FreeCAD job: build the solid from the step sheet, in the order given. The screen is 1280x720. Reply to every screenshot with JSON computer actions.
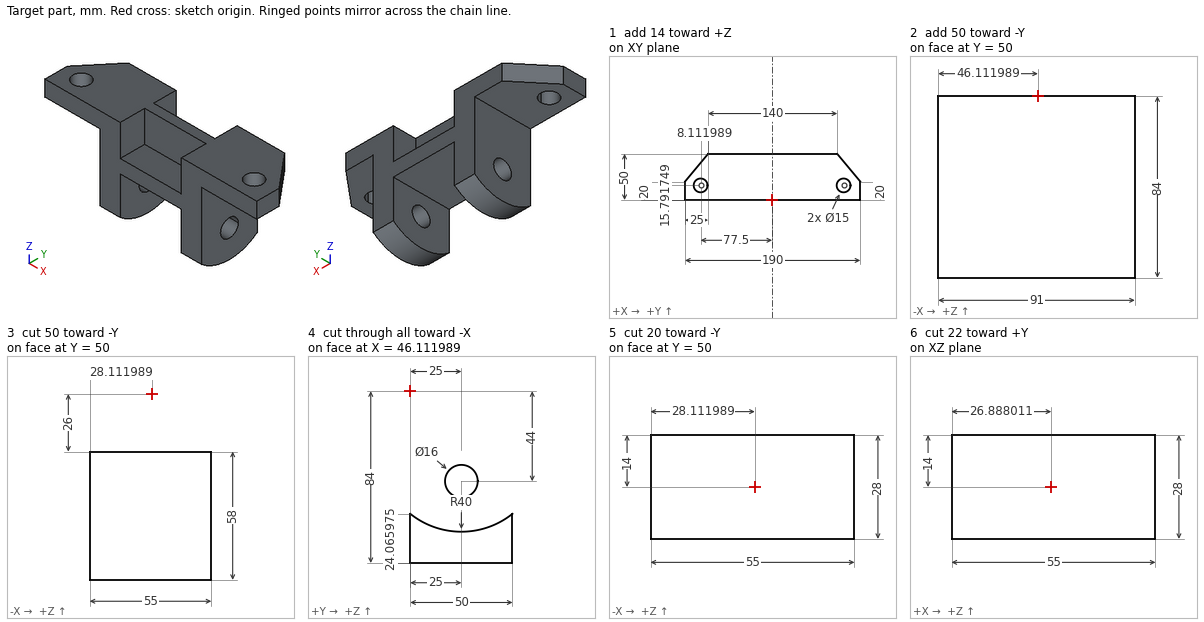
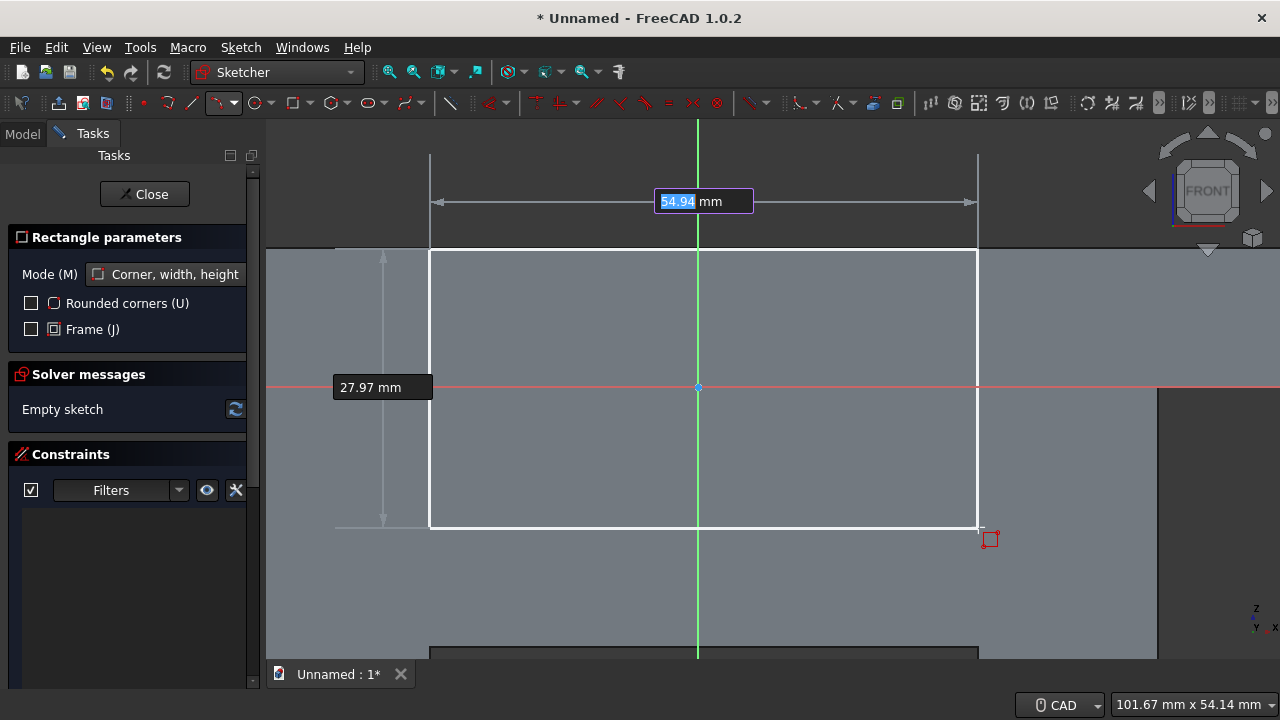
{"action": "type", "text": "55"}
{"action": "key", "text": "Tab"}
{"action": "type", "text": "28"}
{"action": "key", "text": "Return"}
{"action": "key", "text": "Escape"}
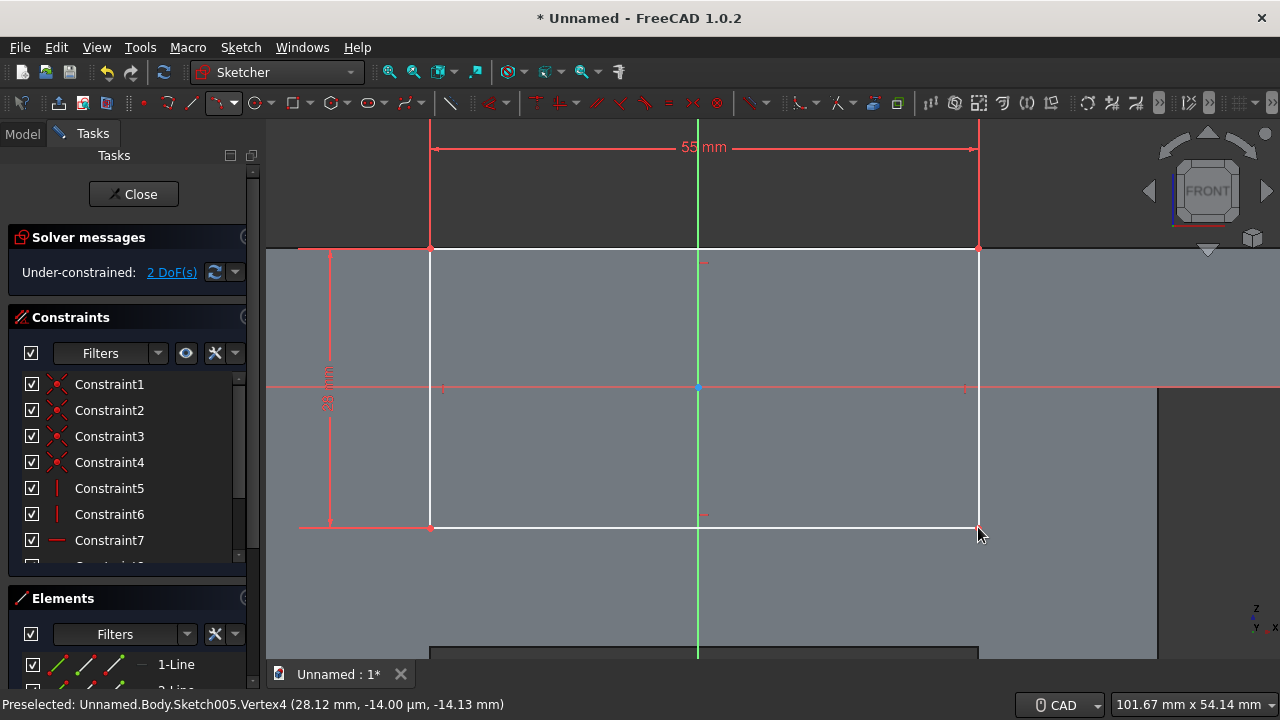
{"action": "left_click", "coordinate": [490, 104]}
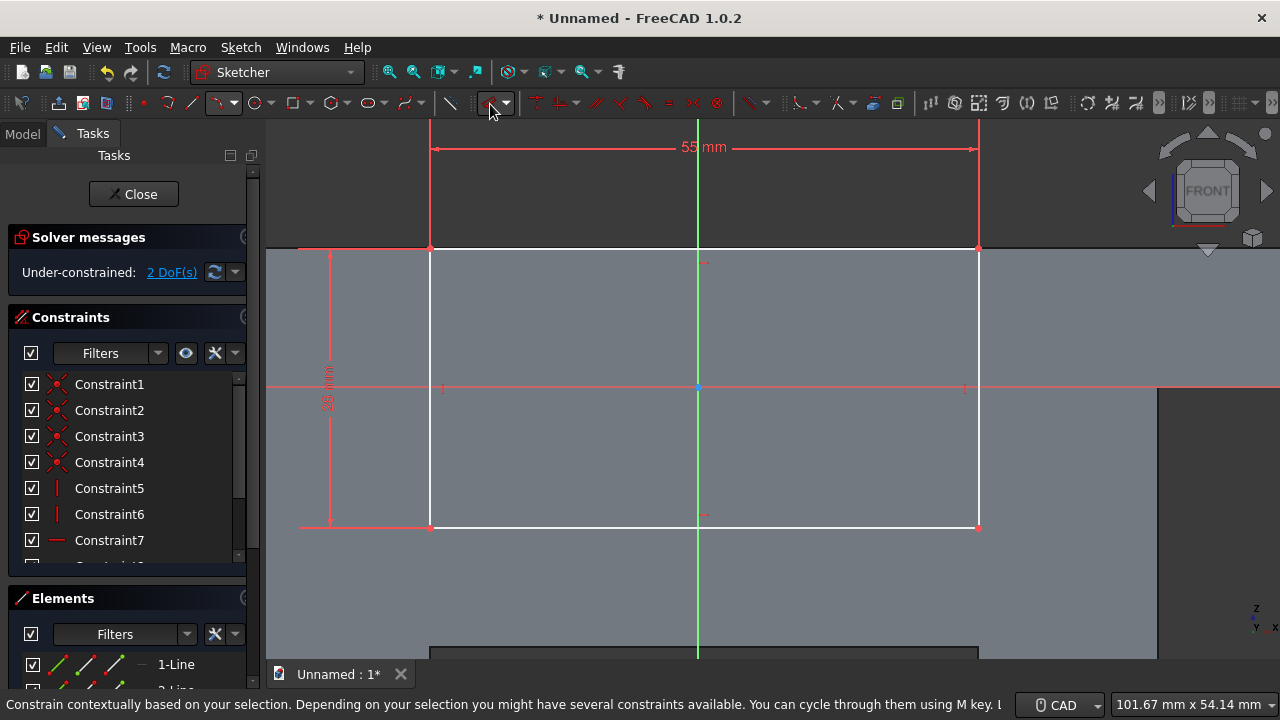
{"action": "left_click", "coordinate": [430, 249]}
{"action": "left_click", "coordinate": [396, 318]}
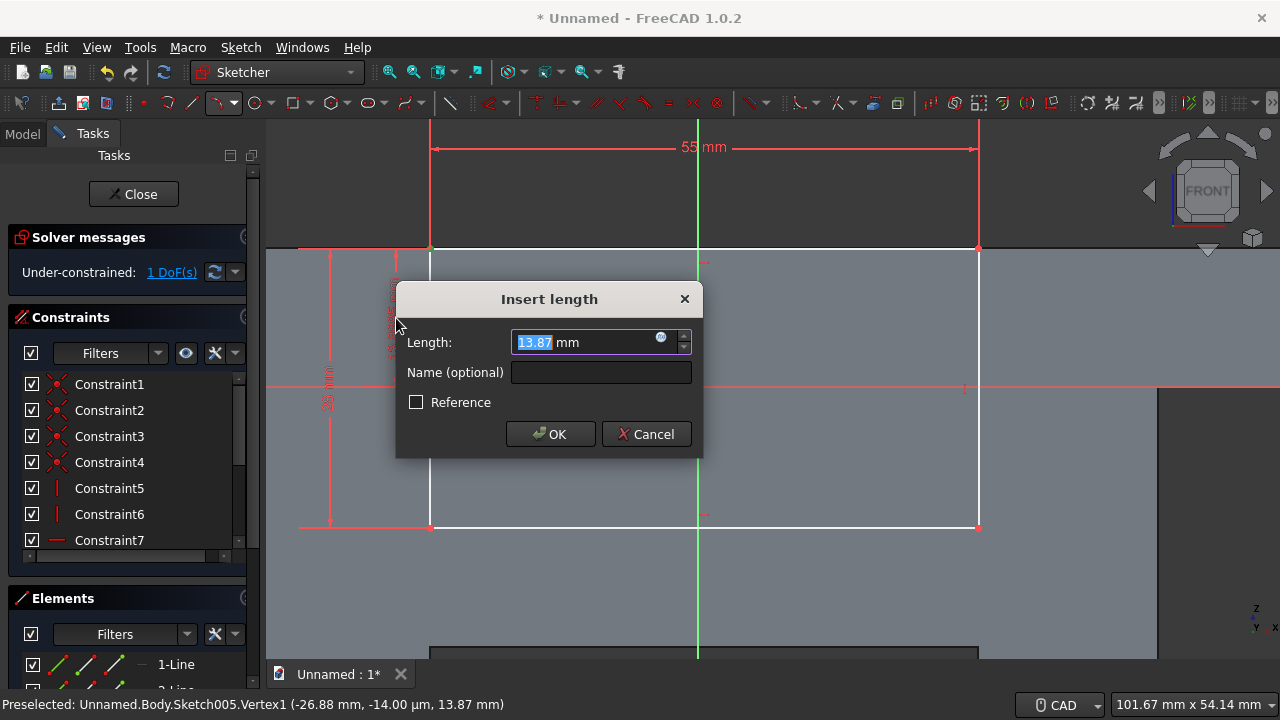
{"action": "type", "text": "14"}
{"action": "key", "text": "Return"}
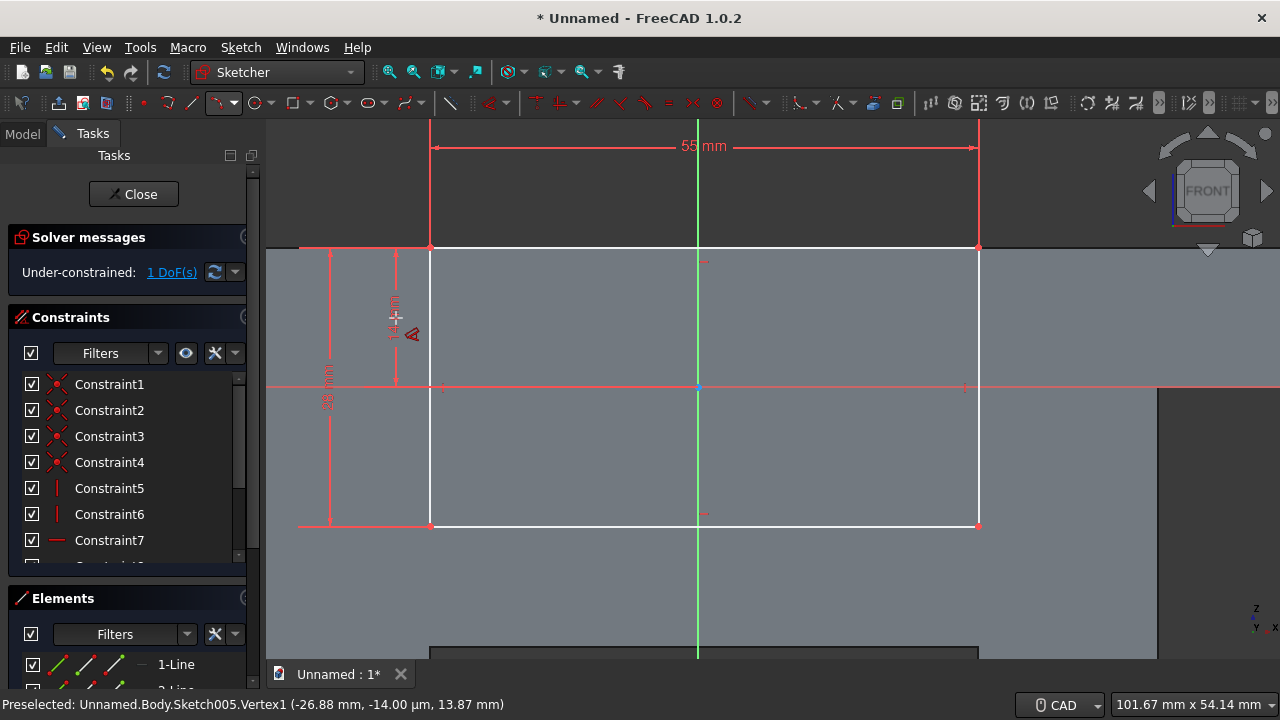
{"action": "left_click", "coordinate": [430, 248]}
{"action": "left_click", "coordinate": [564, 214]}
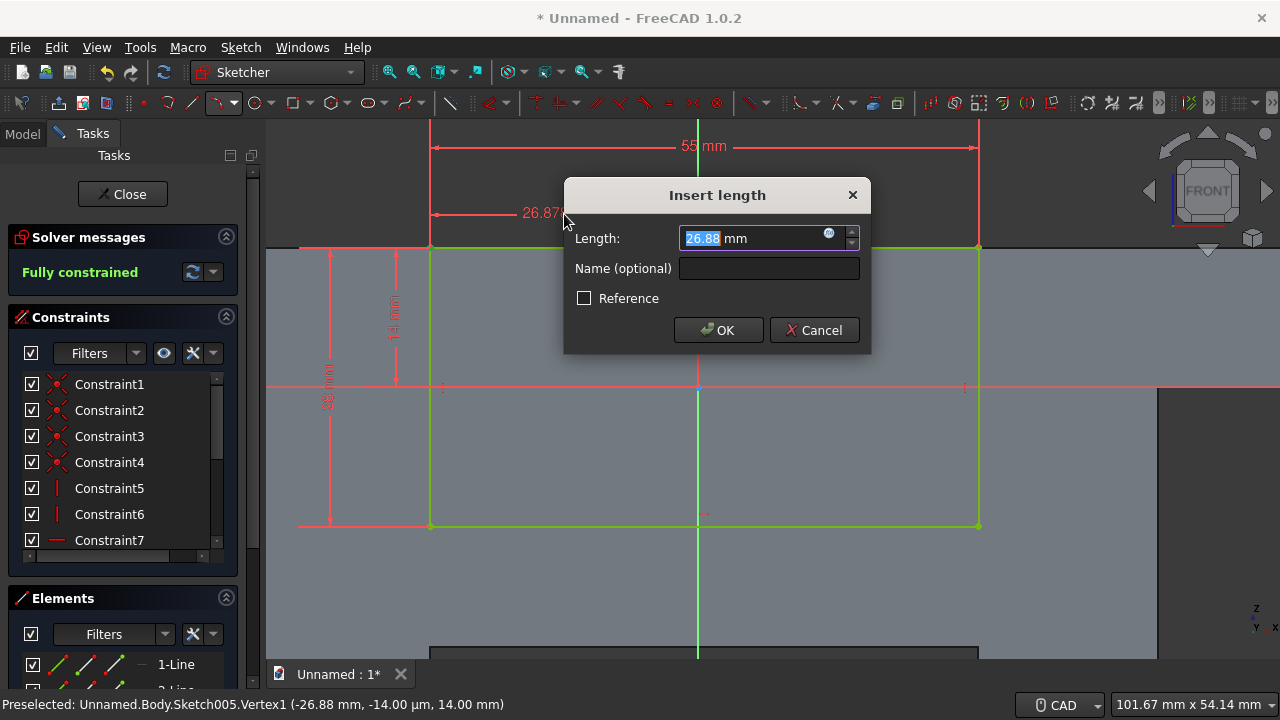
{"action": "type", "text": "26.888011"}
{"action": "key", "text": "Return"}
{"action": "key", "text": "Escape"}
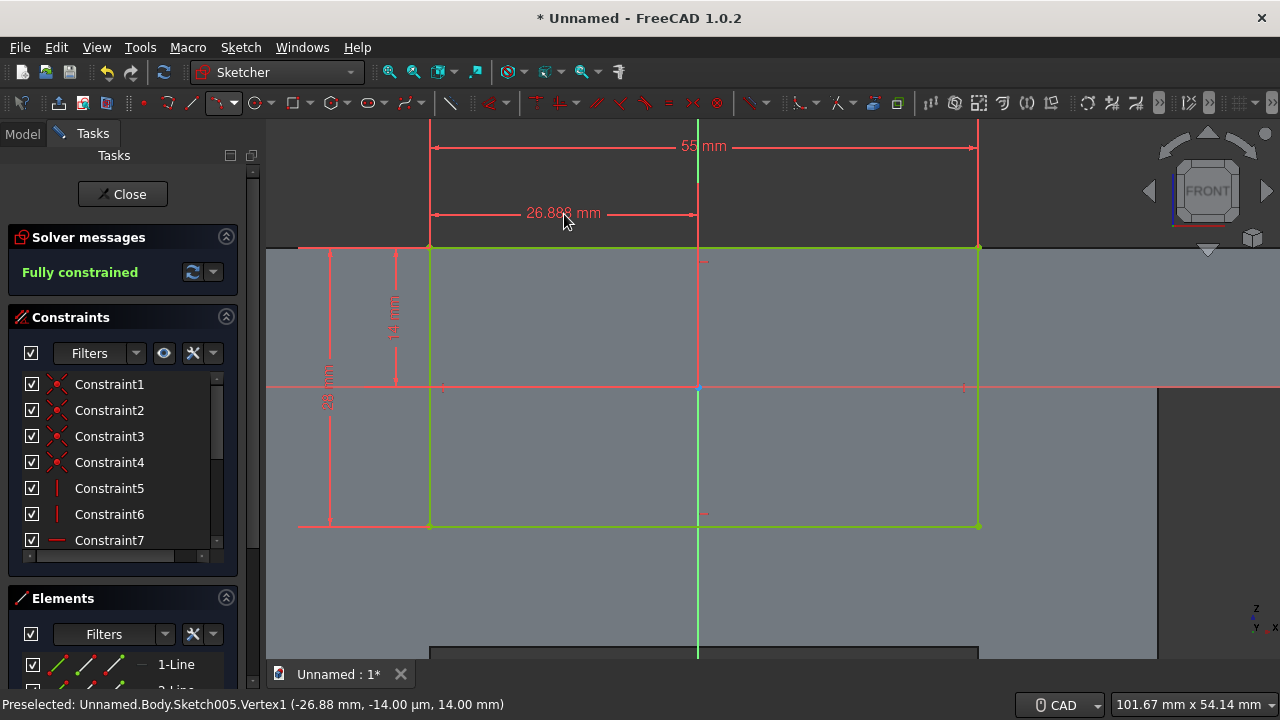
{"action": "left_click", "coordinate": [123, 194]}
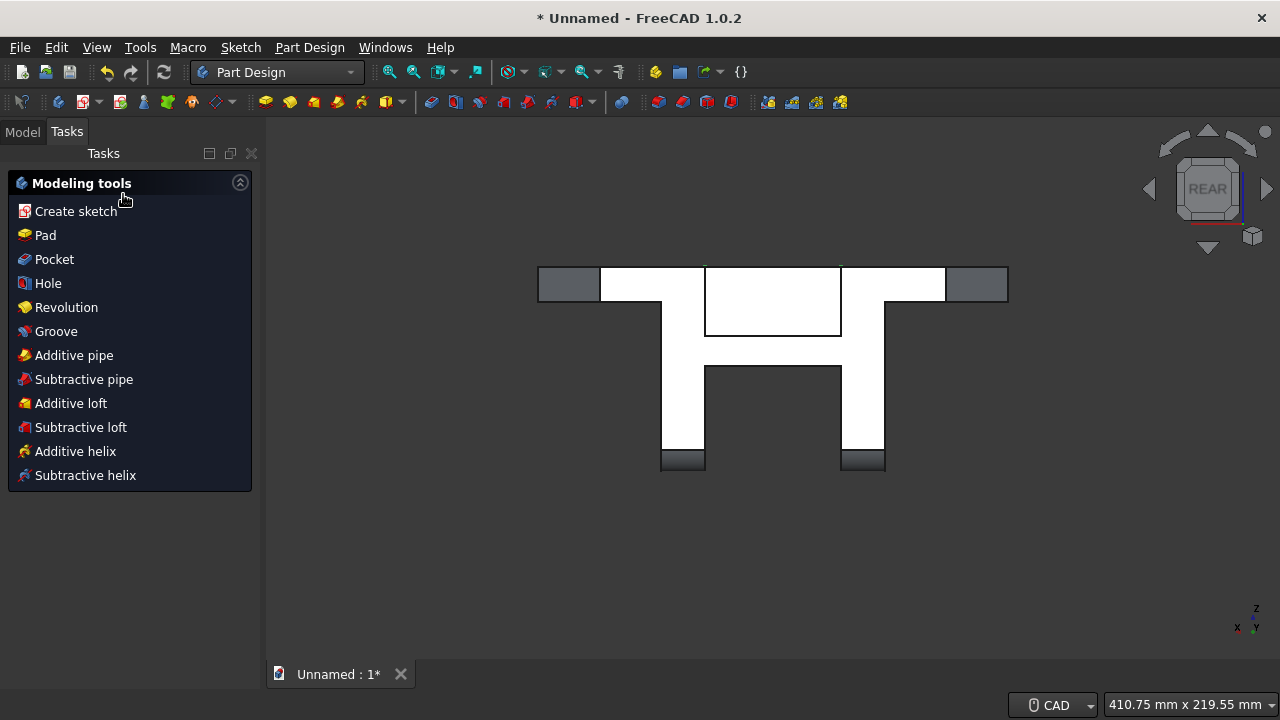
{"action": "left_click", "coordinate": [432, 102]}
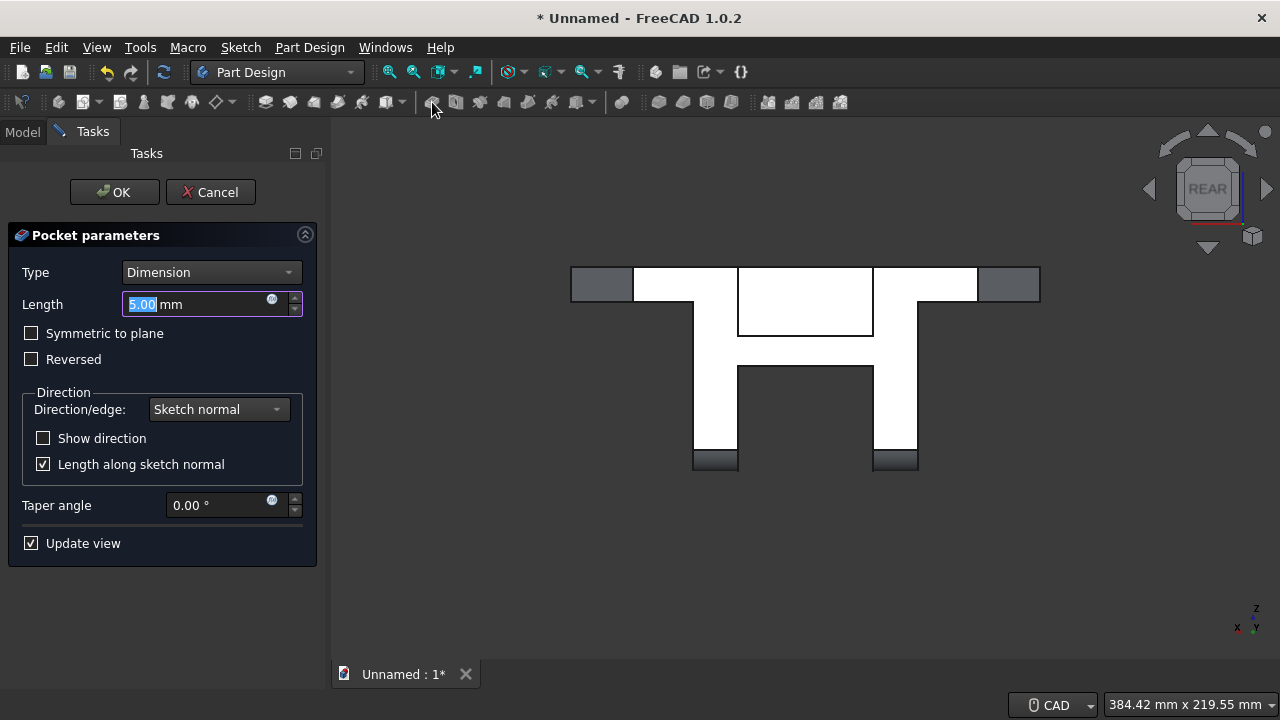
{"action": "type", "text": "22"}
{"action": "key", "text": "Tab"}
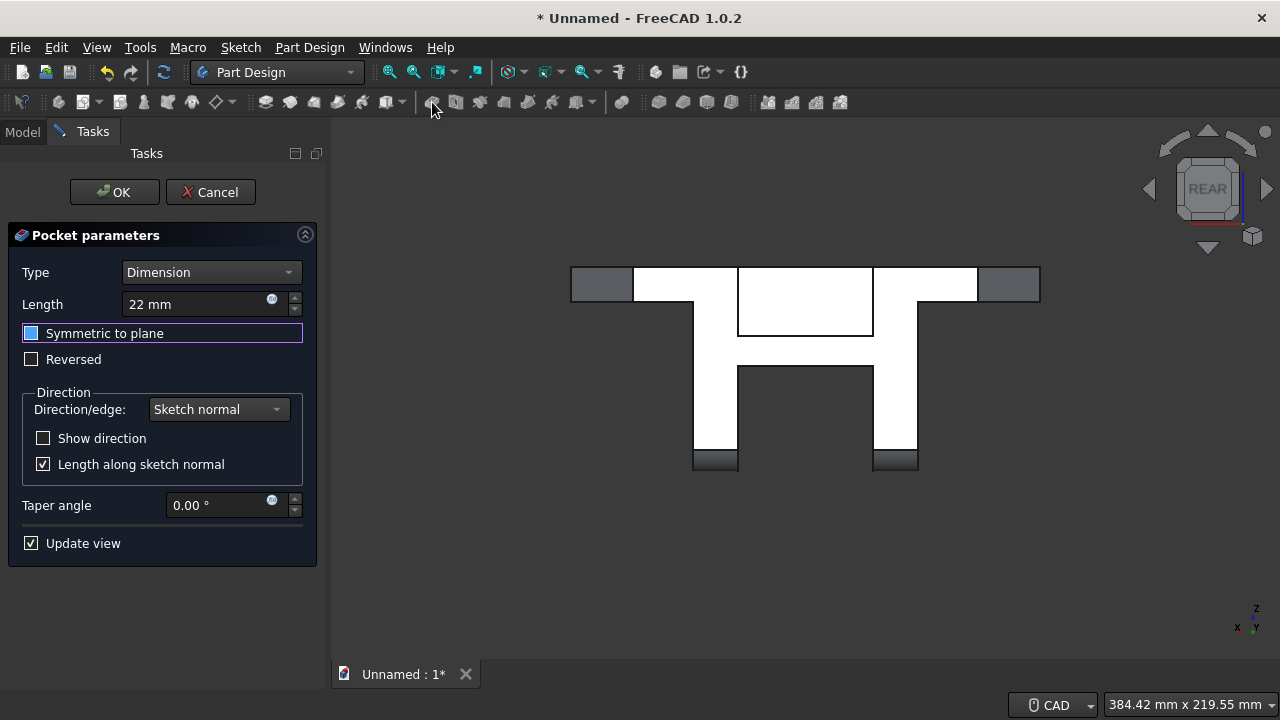
{"action": "left_click", "coordinate": [115, 192]}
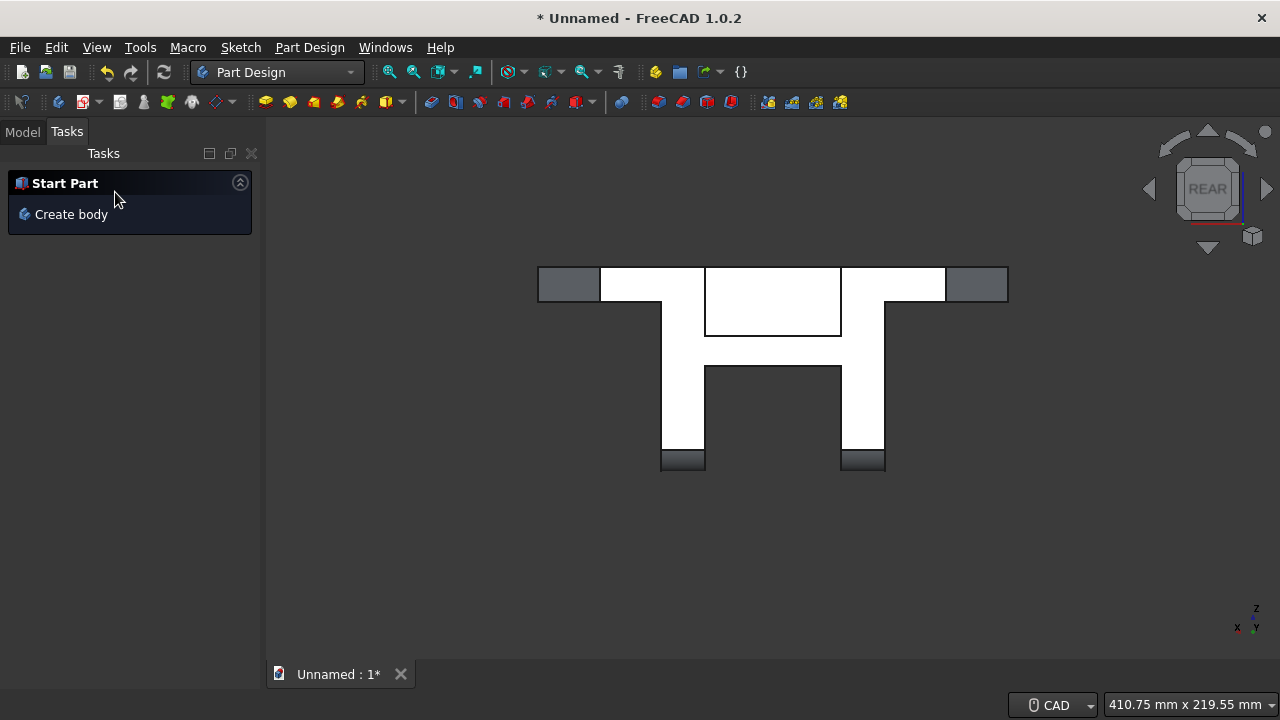
{"action": "key", "text": "0"}